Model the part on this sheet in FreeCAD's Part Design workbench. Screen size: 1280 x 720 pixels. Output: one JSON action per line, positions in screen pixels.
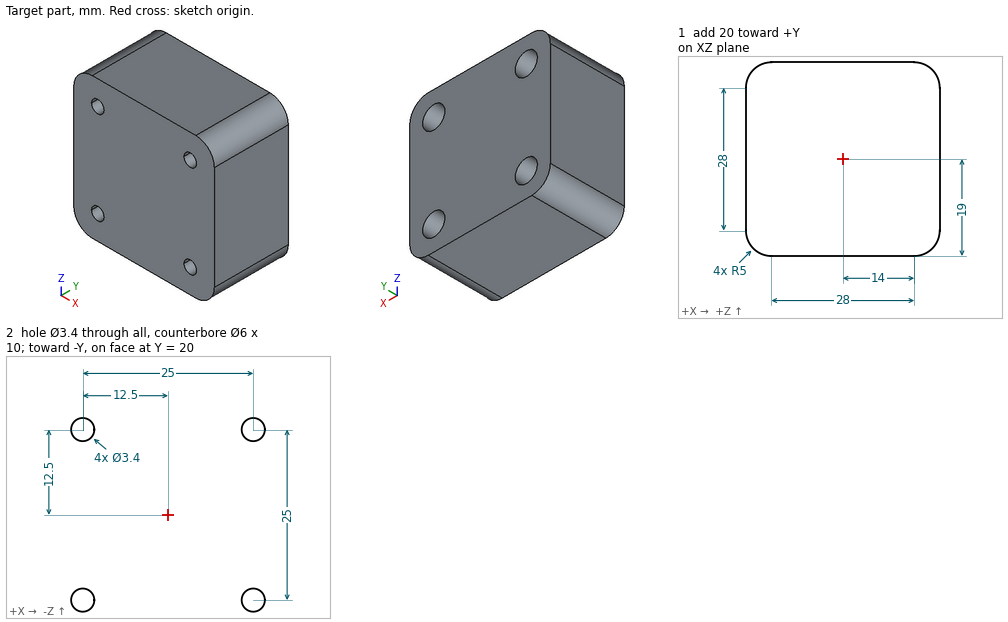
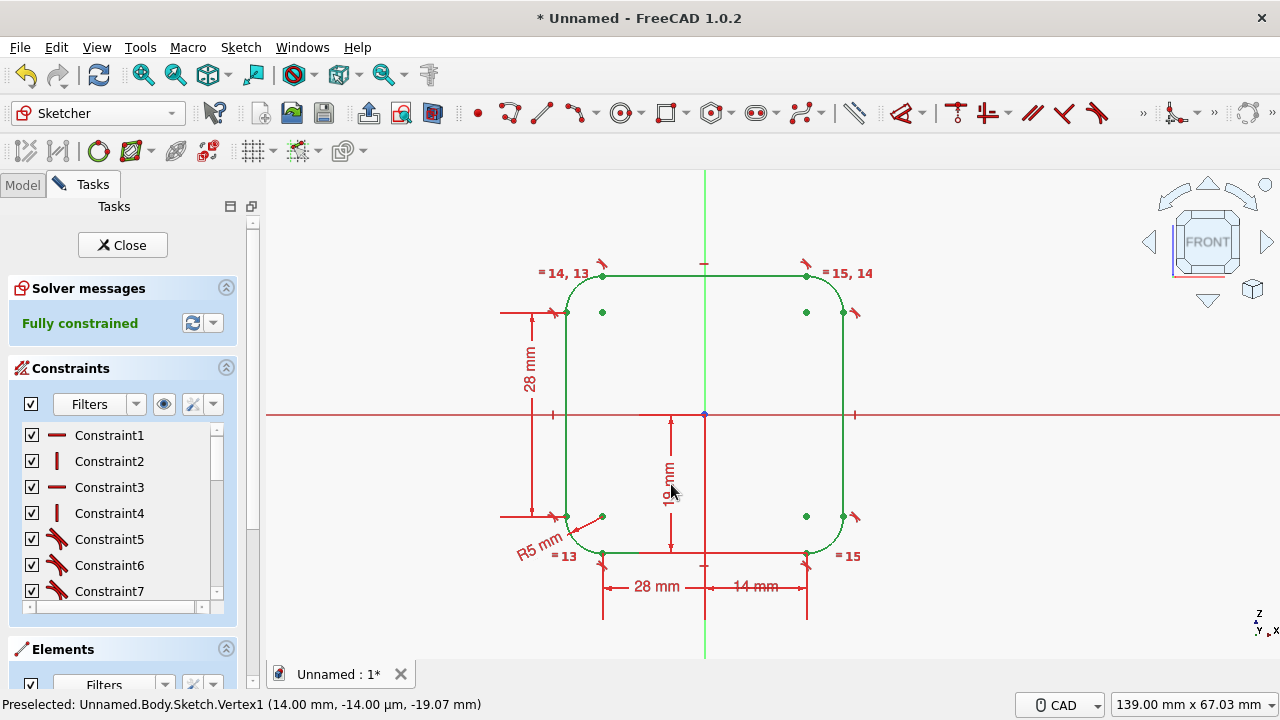
{"action": "left_click", "coordinate": [123, 245]}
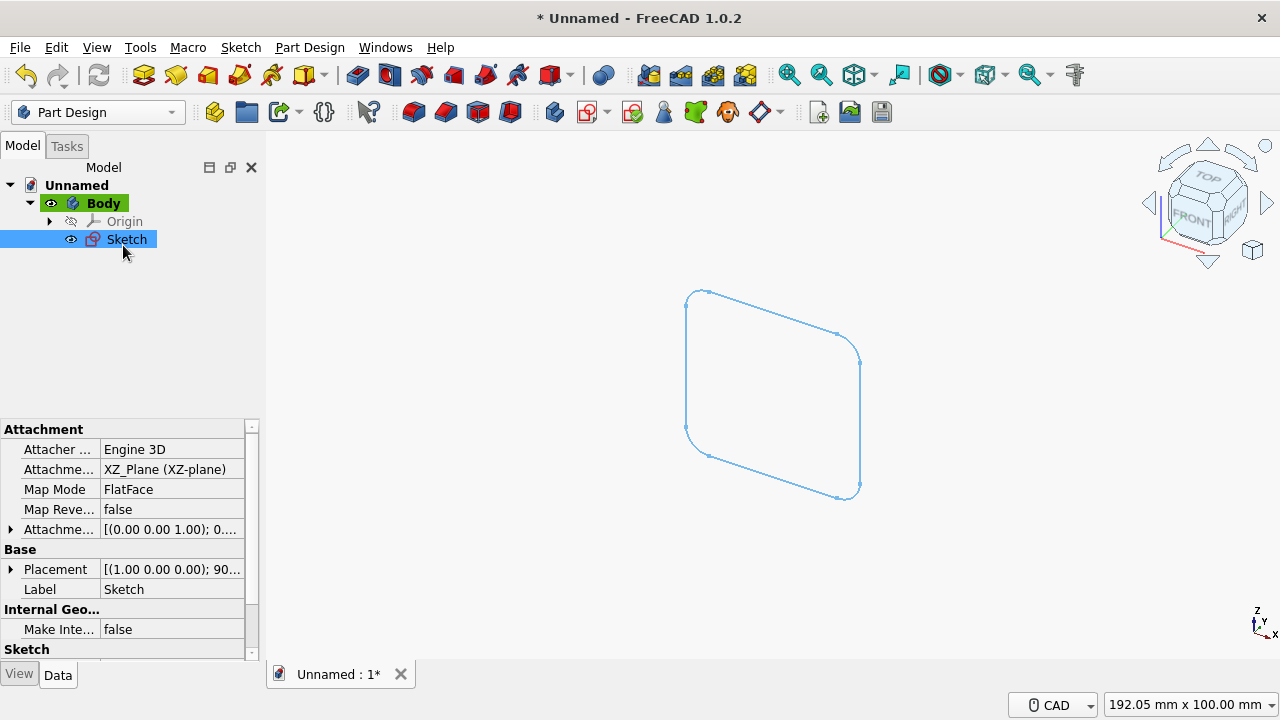
{"action": "left_click", "coordinate": [144, 76]}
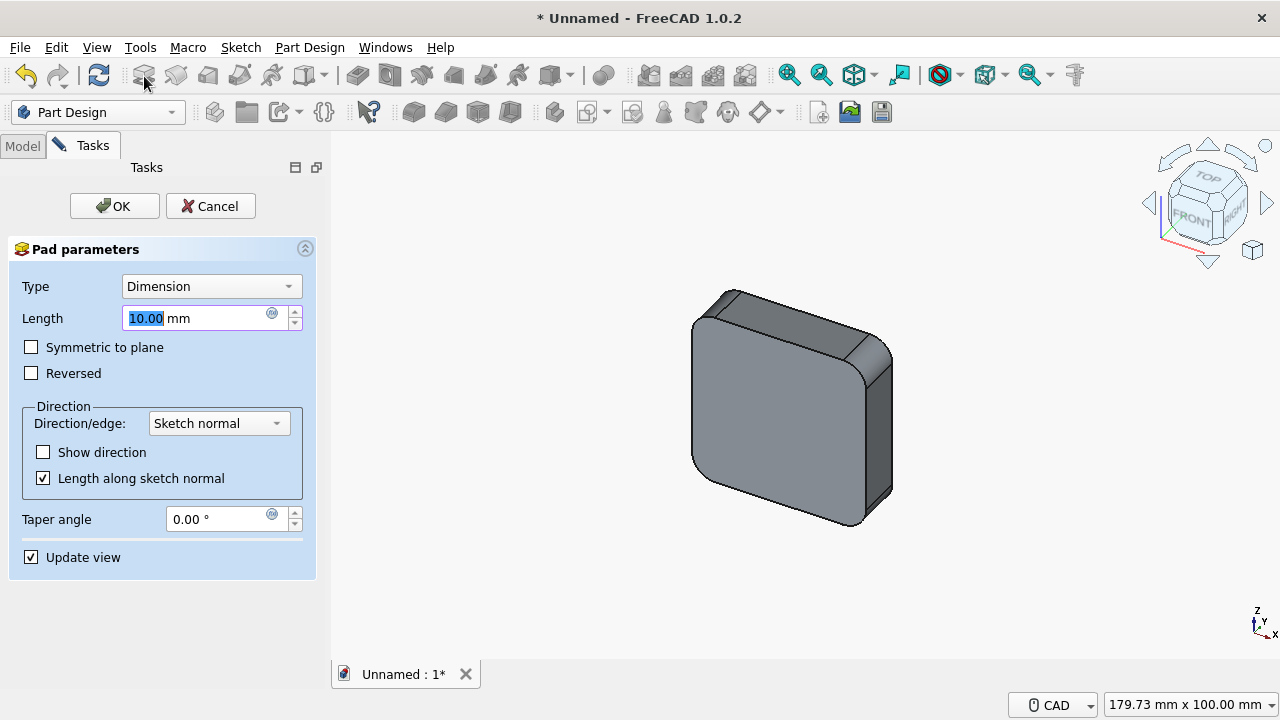
{"action": "type", "text": "20"}
{"action": "key", "text": "Tab"}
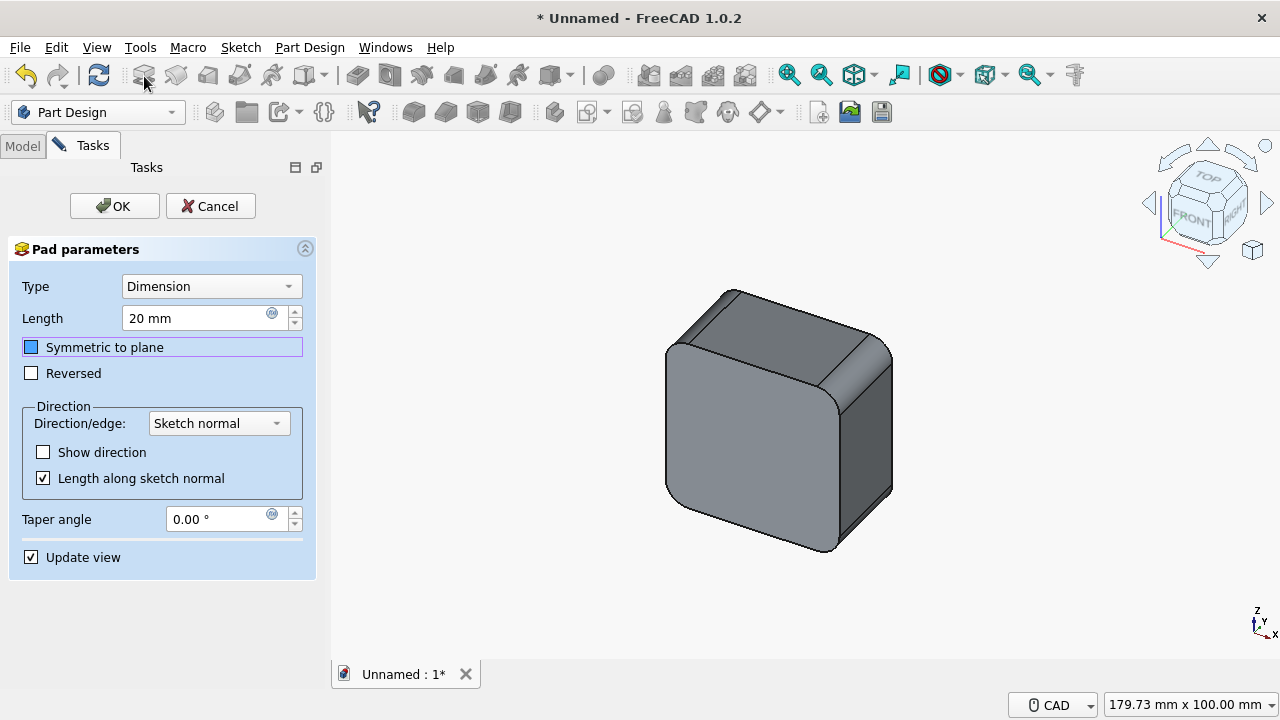
{"action": "left_click", "coordinate": [30, 373]}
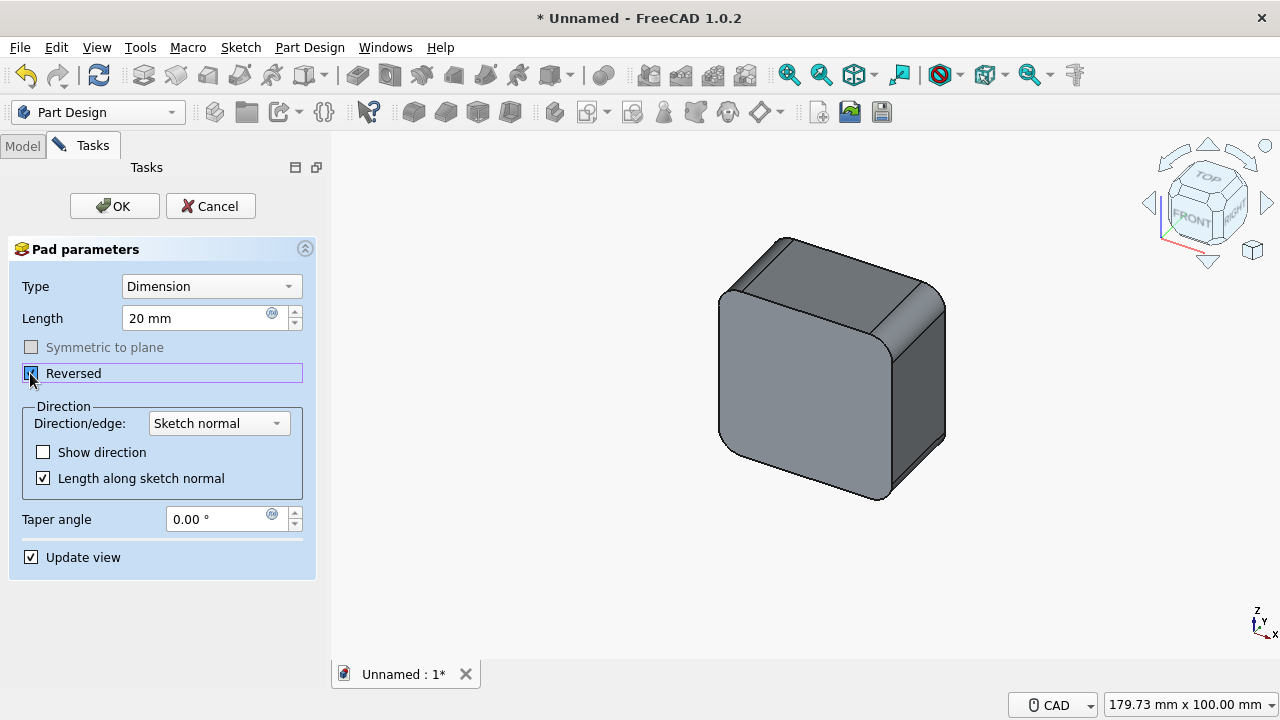
{"action": "left_click", "coordinate": [115, 206]}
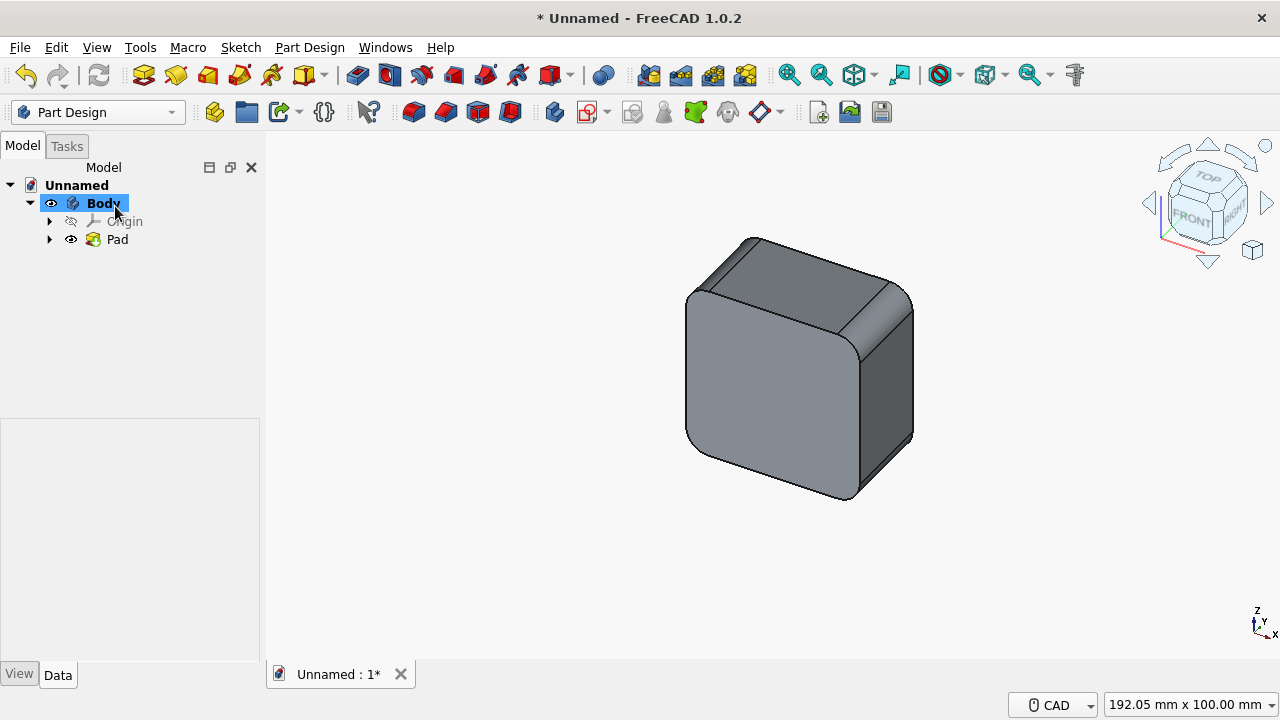
{"action": "key", "text": "4"}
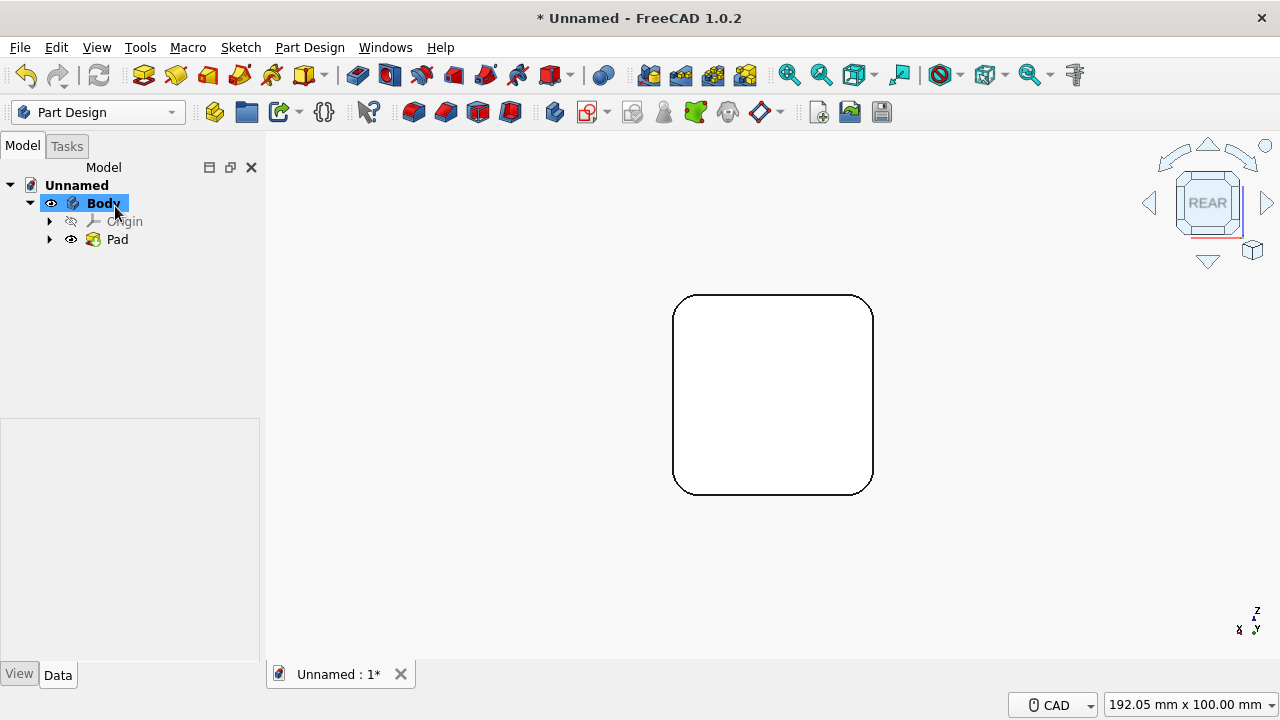
{"action": "left_click", "coordinate": [790, 76]}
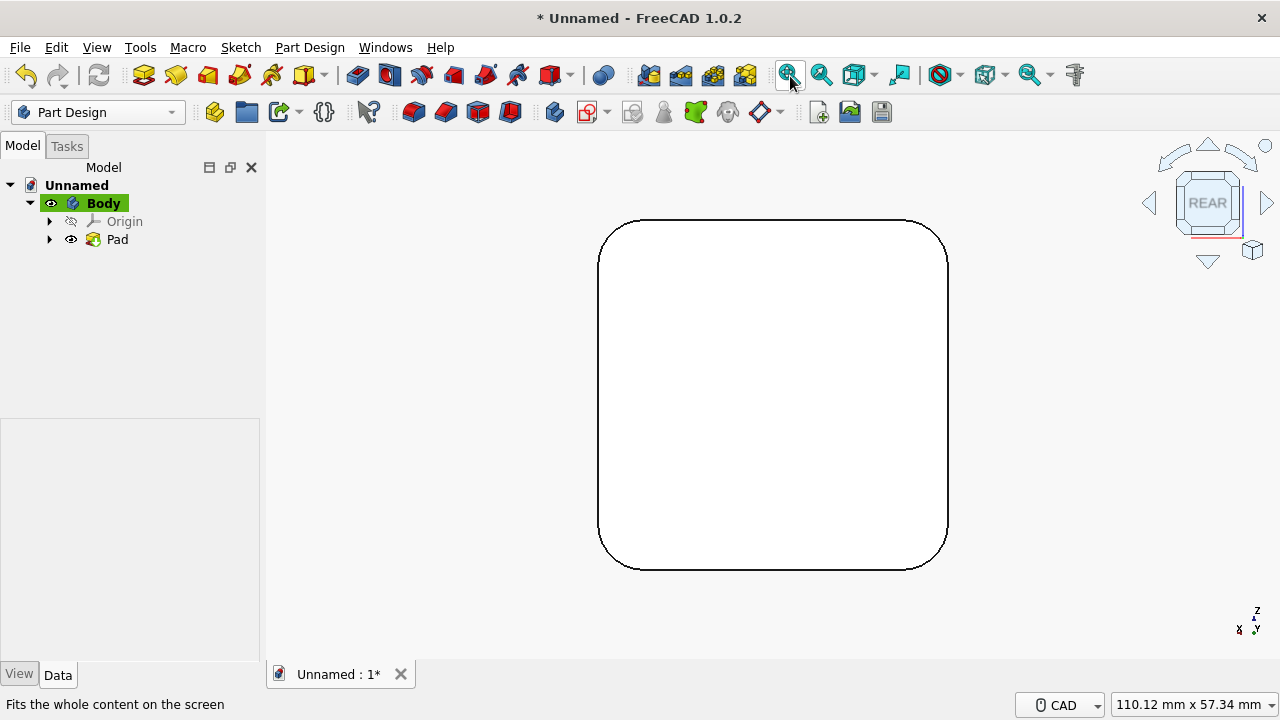
{"action": "left_click", "coordinate": [773, 394]}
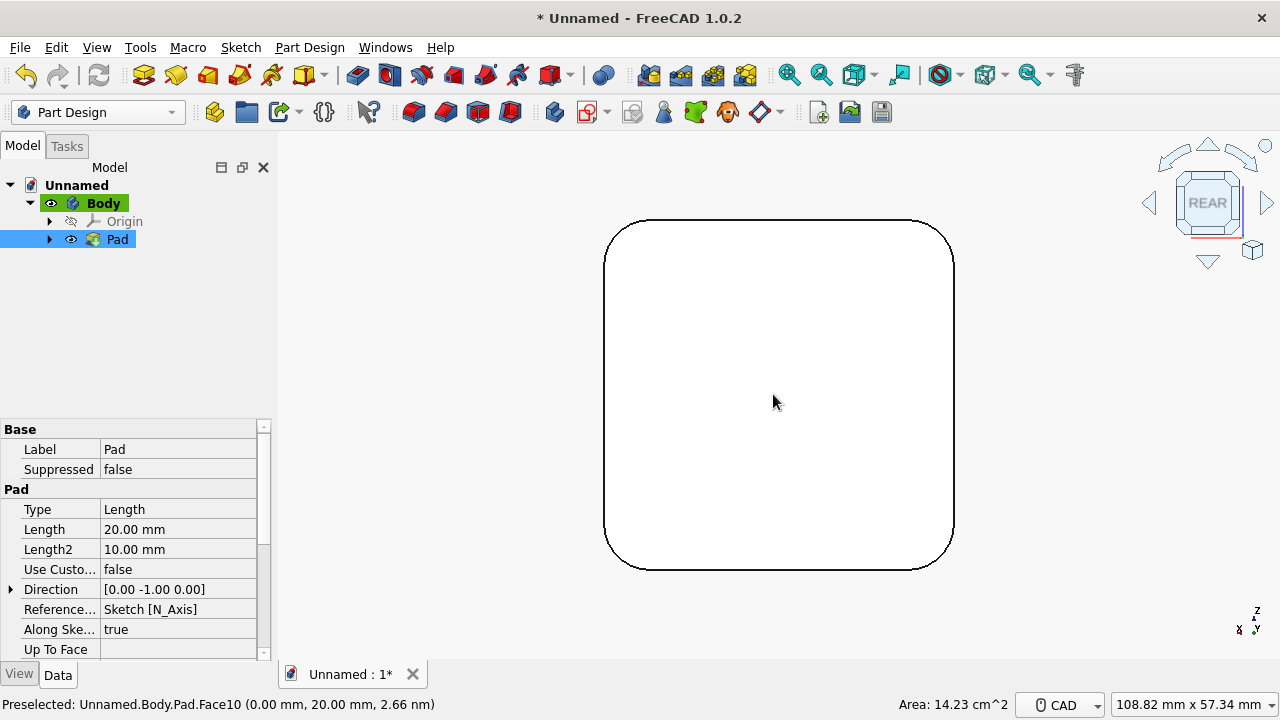
{"action": "left_click", "coordinate": [588, 112]}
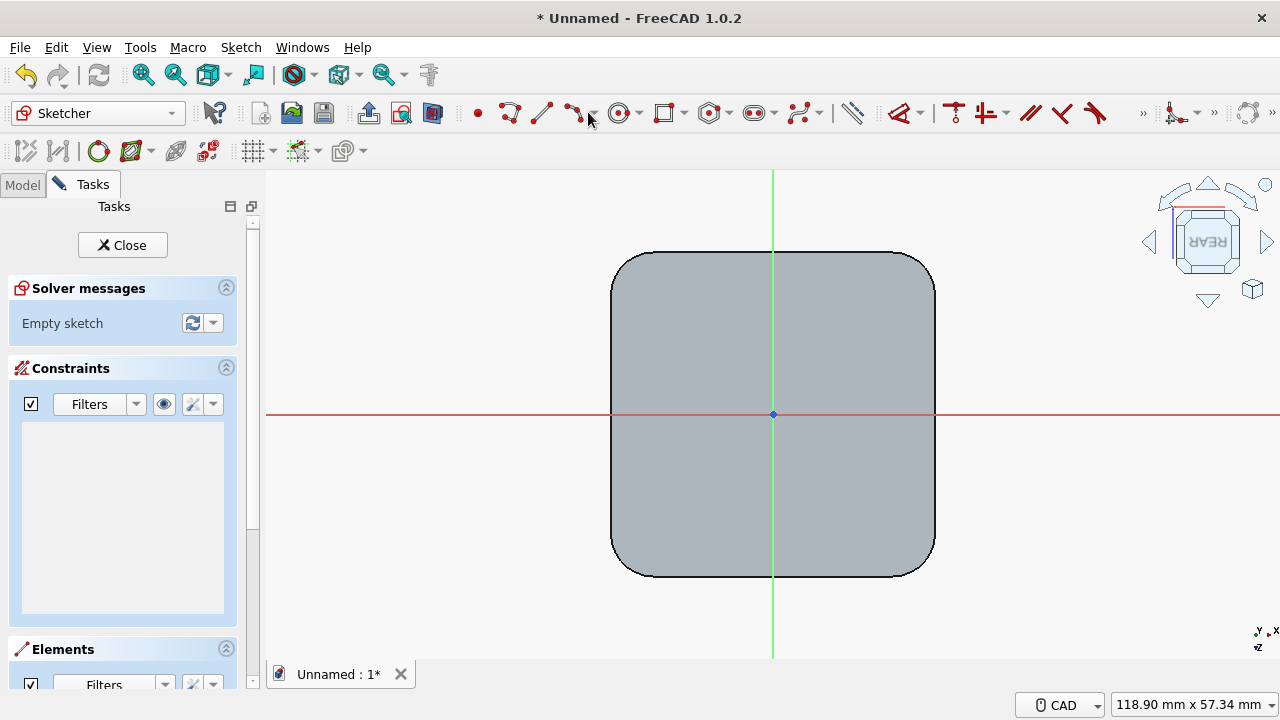
{"action": "left_click", "coordinate": [620, 114]}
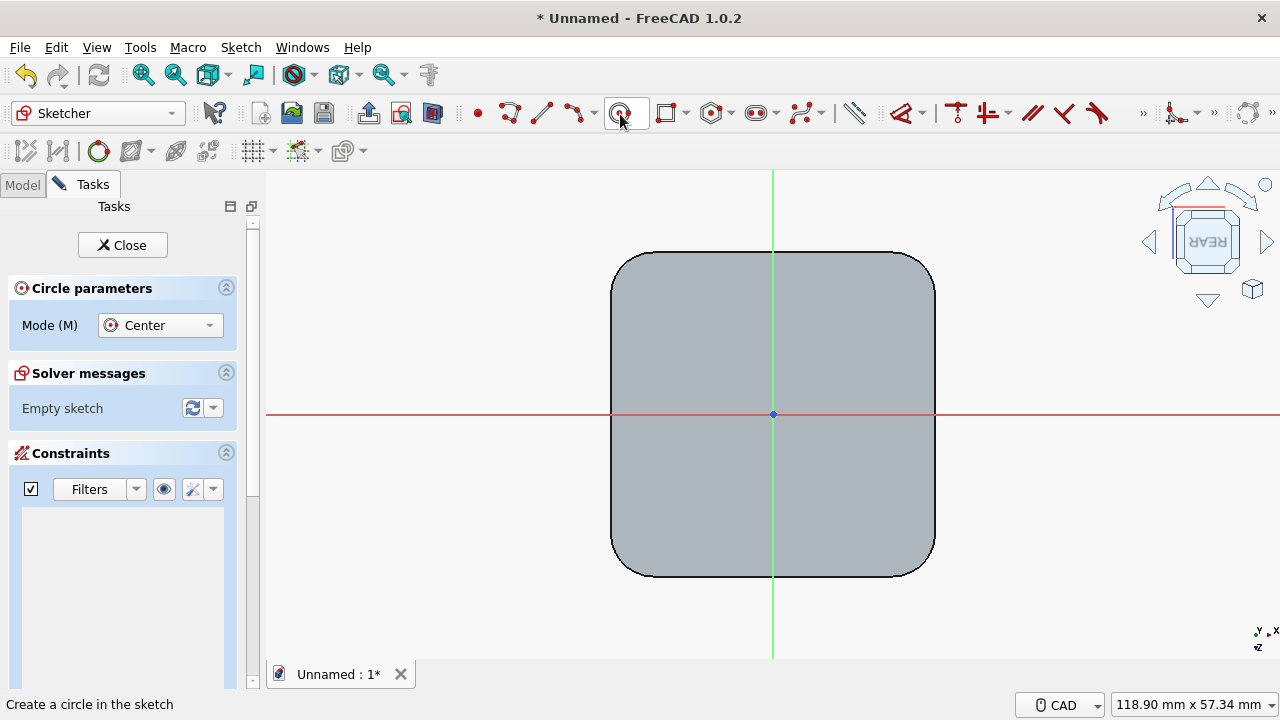
{"action": "scroll", "coordinate": [666, 308], "scroll_direction": "up", "scroll_amount": 3}